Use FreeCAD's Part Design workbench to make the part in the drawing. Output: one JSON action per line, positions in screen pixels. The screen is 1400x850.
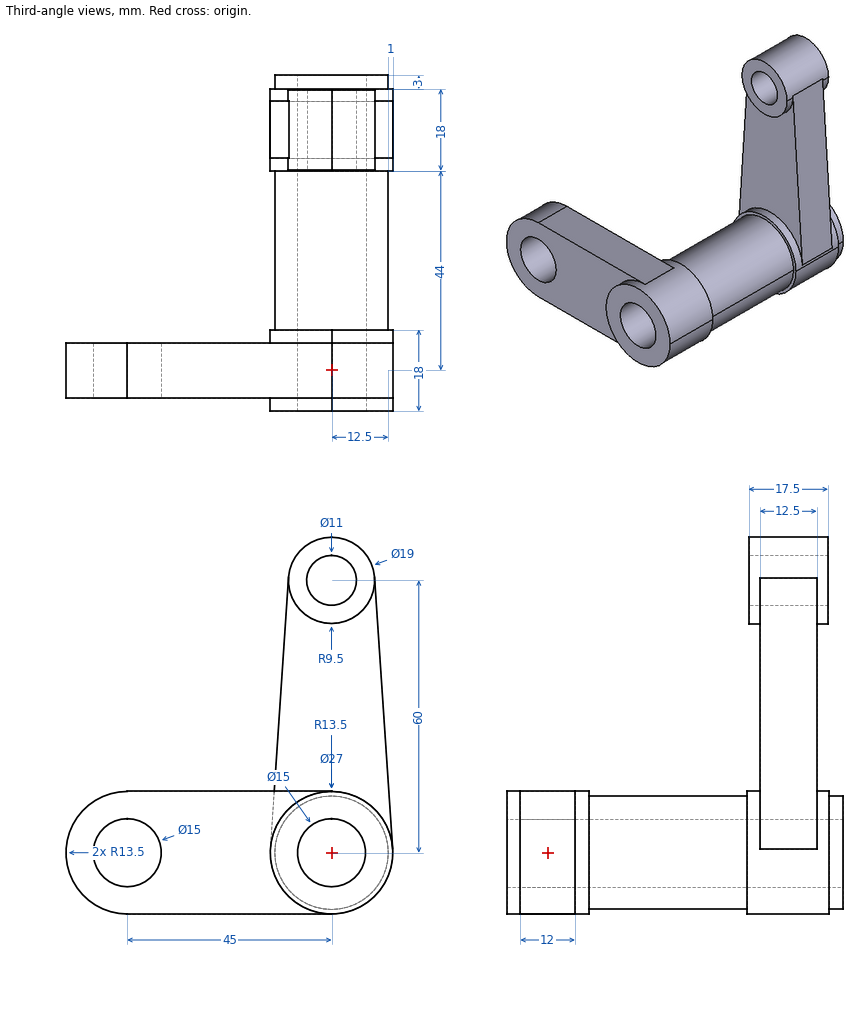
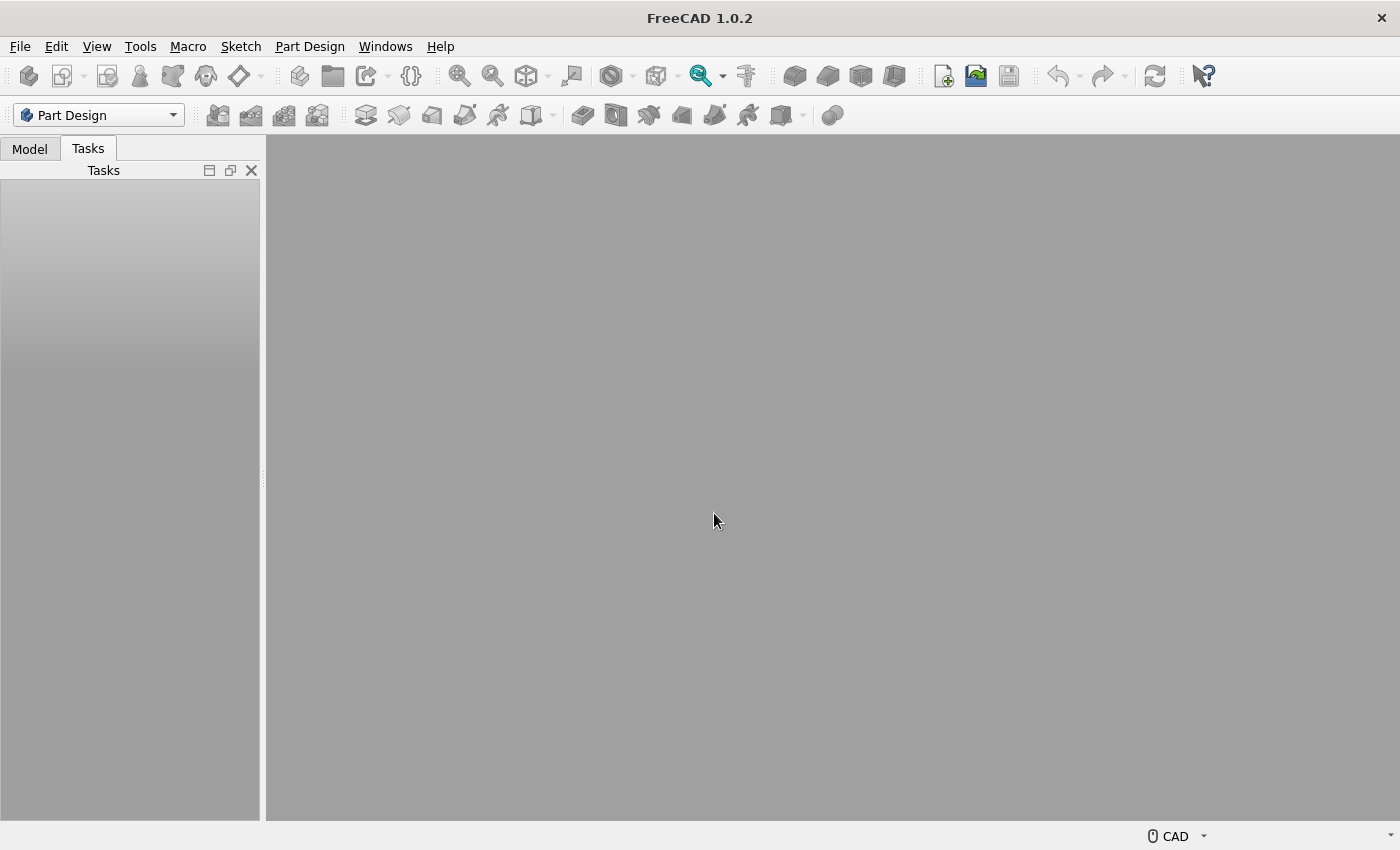
{"action": "left_click", "coordinate": [943, 76]}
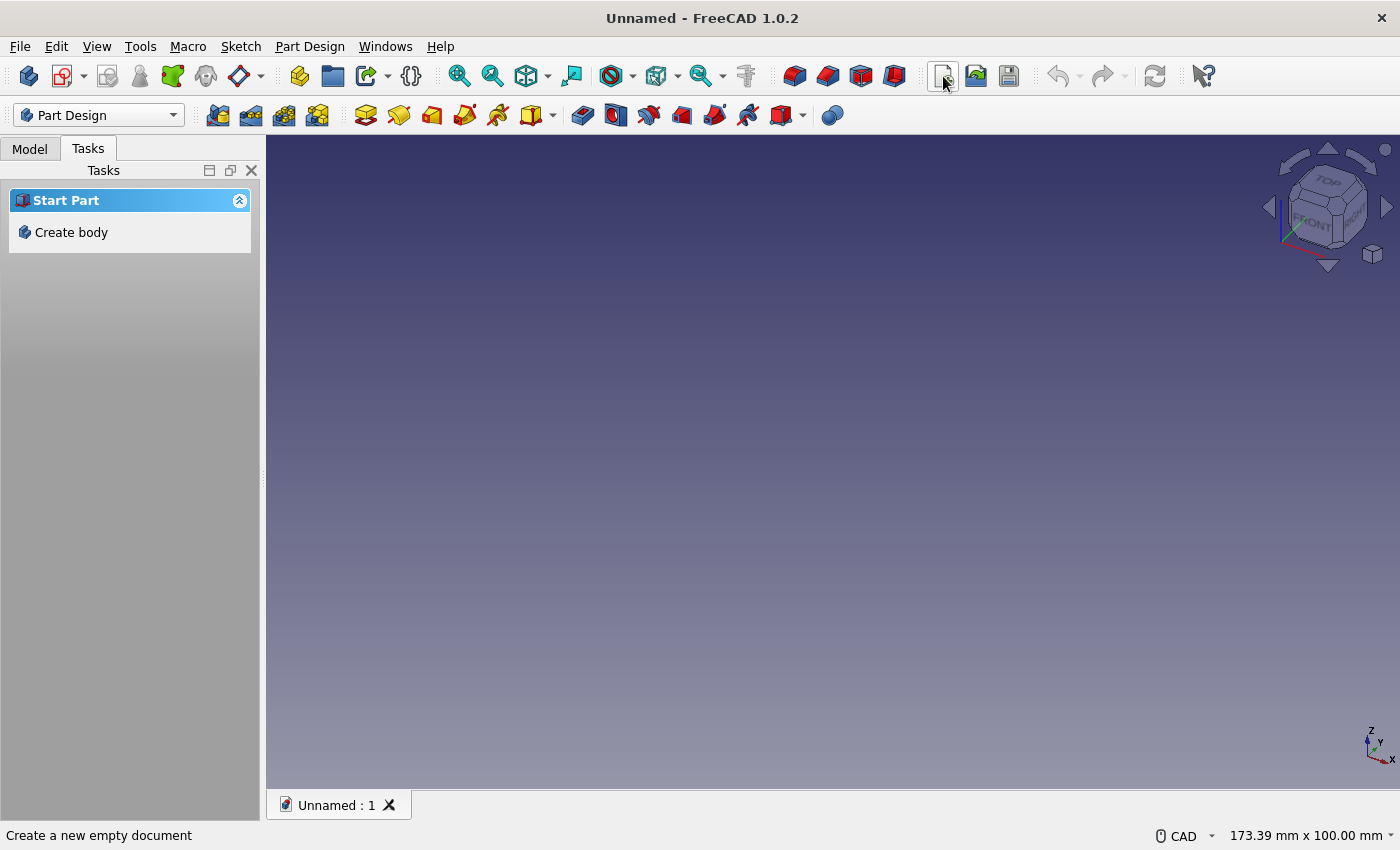
{"action": "left_click", "coordinate": [62, 76]}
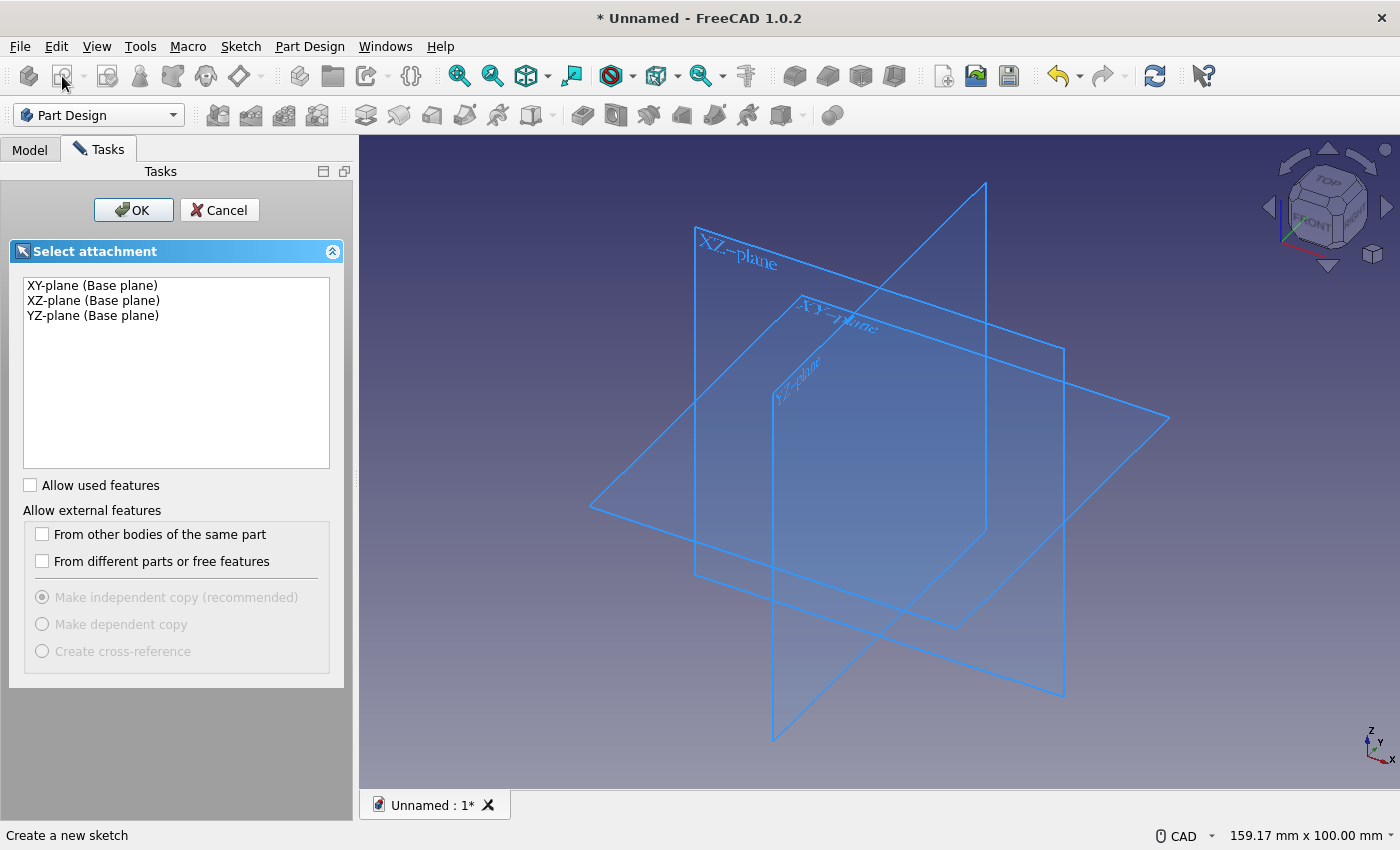
{"action": "left_click", "coordinate": [84, 300]}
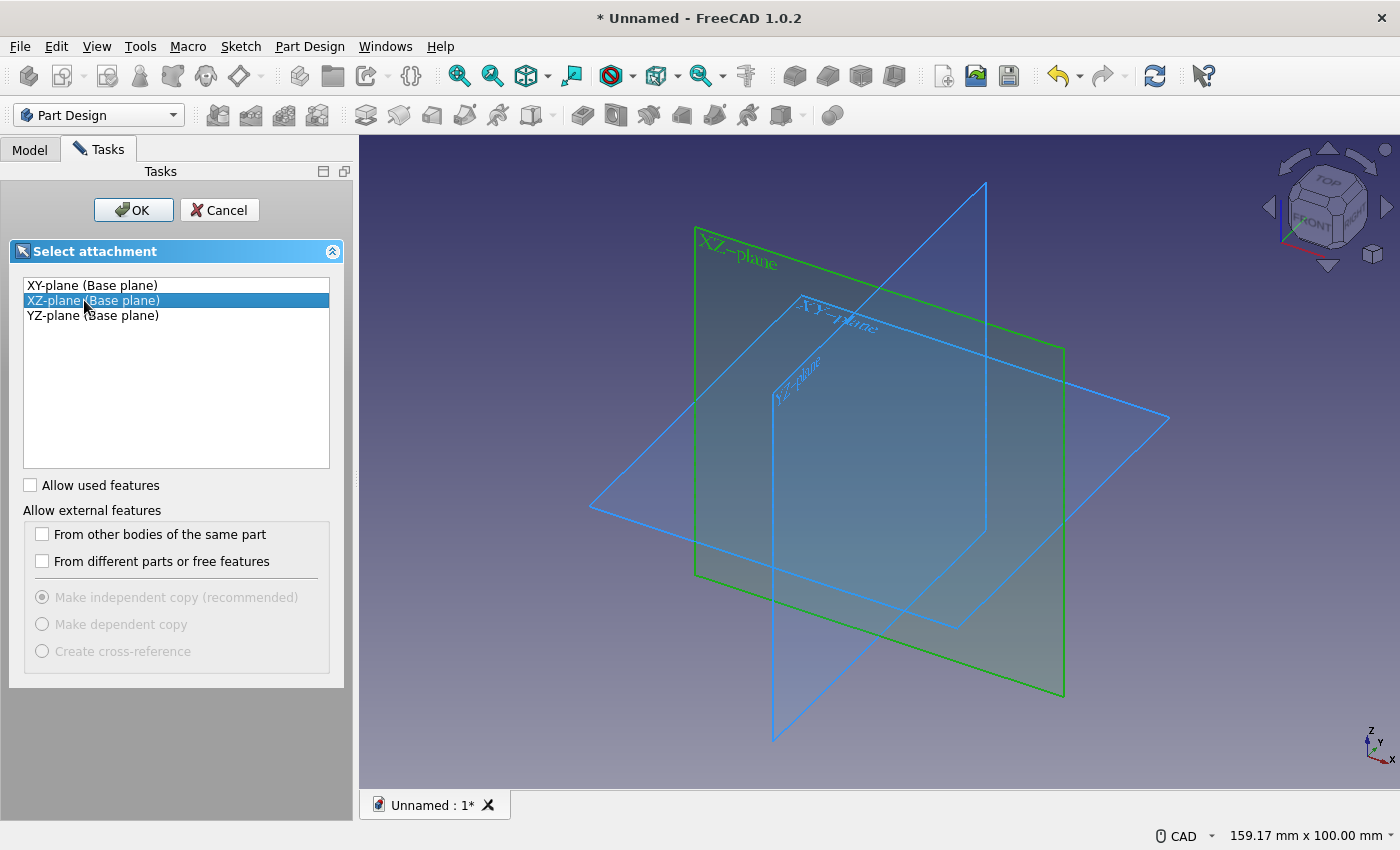
{"action": "left_click", "coordinate": [134, 210]}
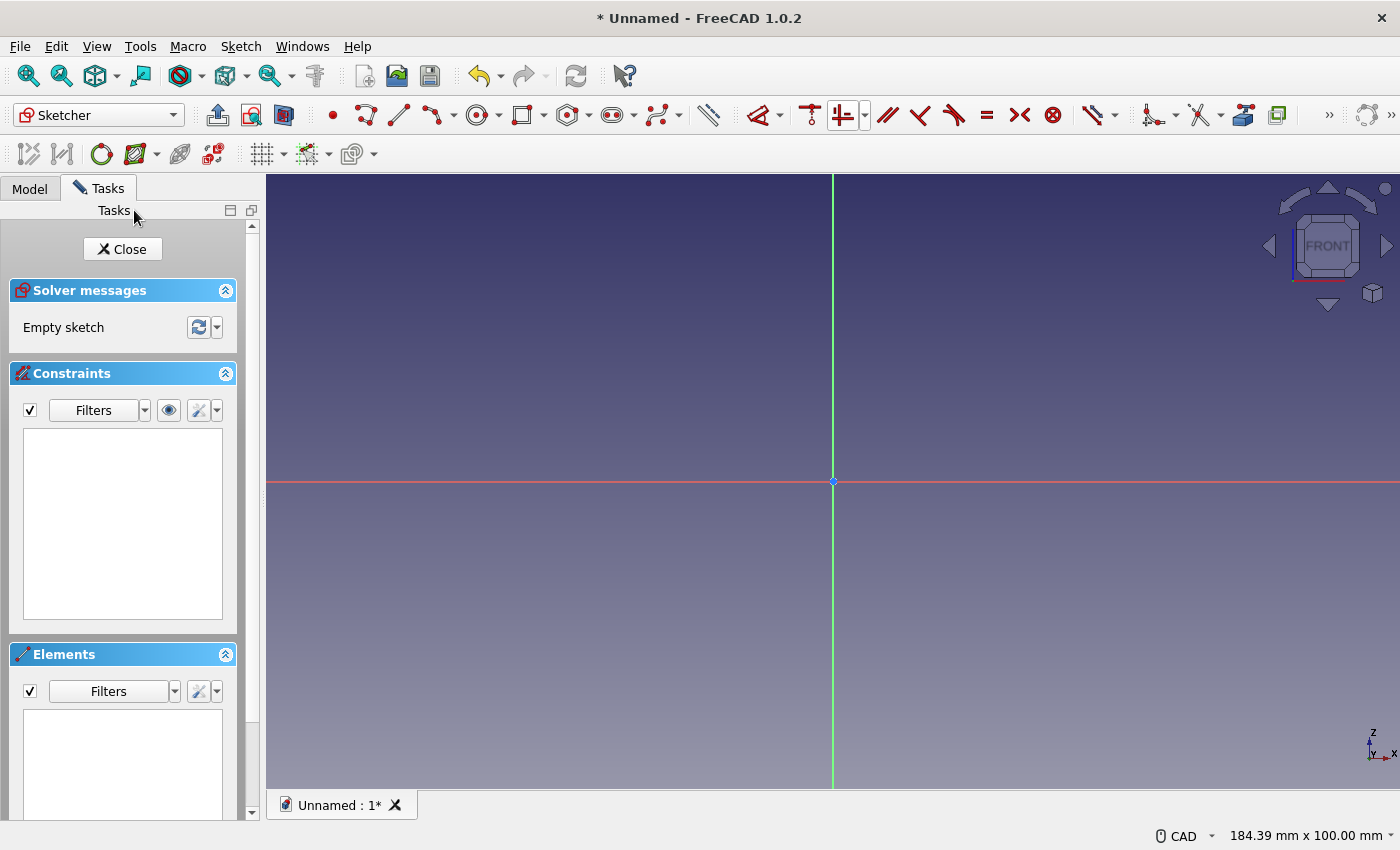
{"action": "scroll", "coordinate": [553, 482], "scroll_direction": "up", "scroll_amount": 2}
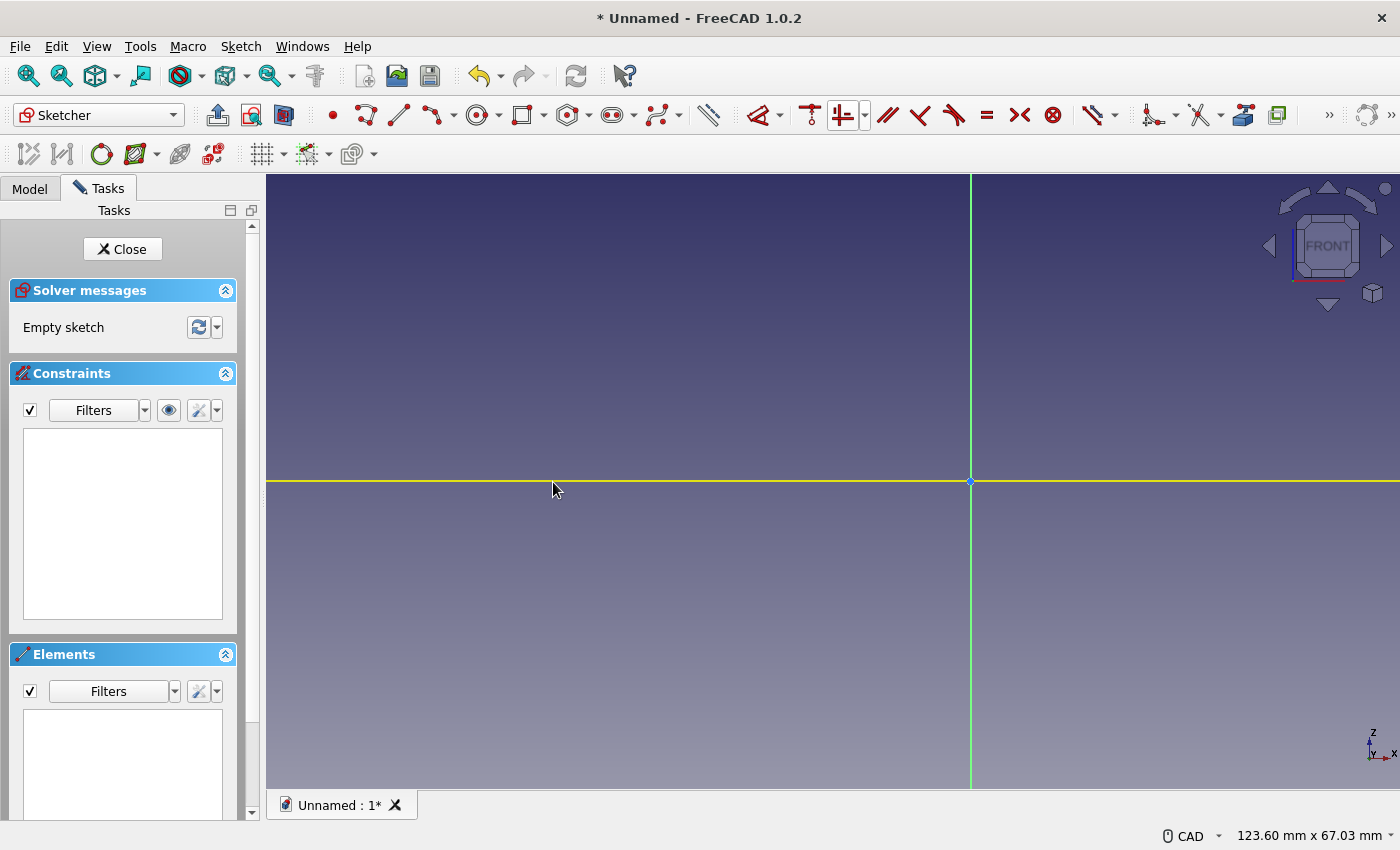
{"action": "key", "text": "g s"}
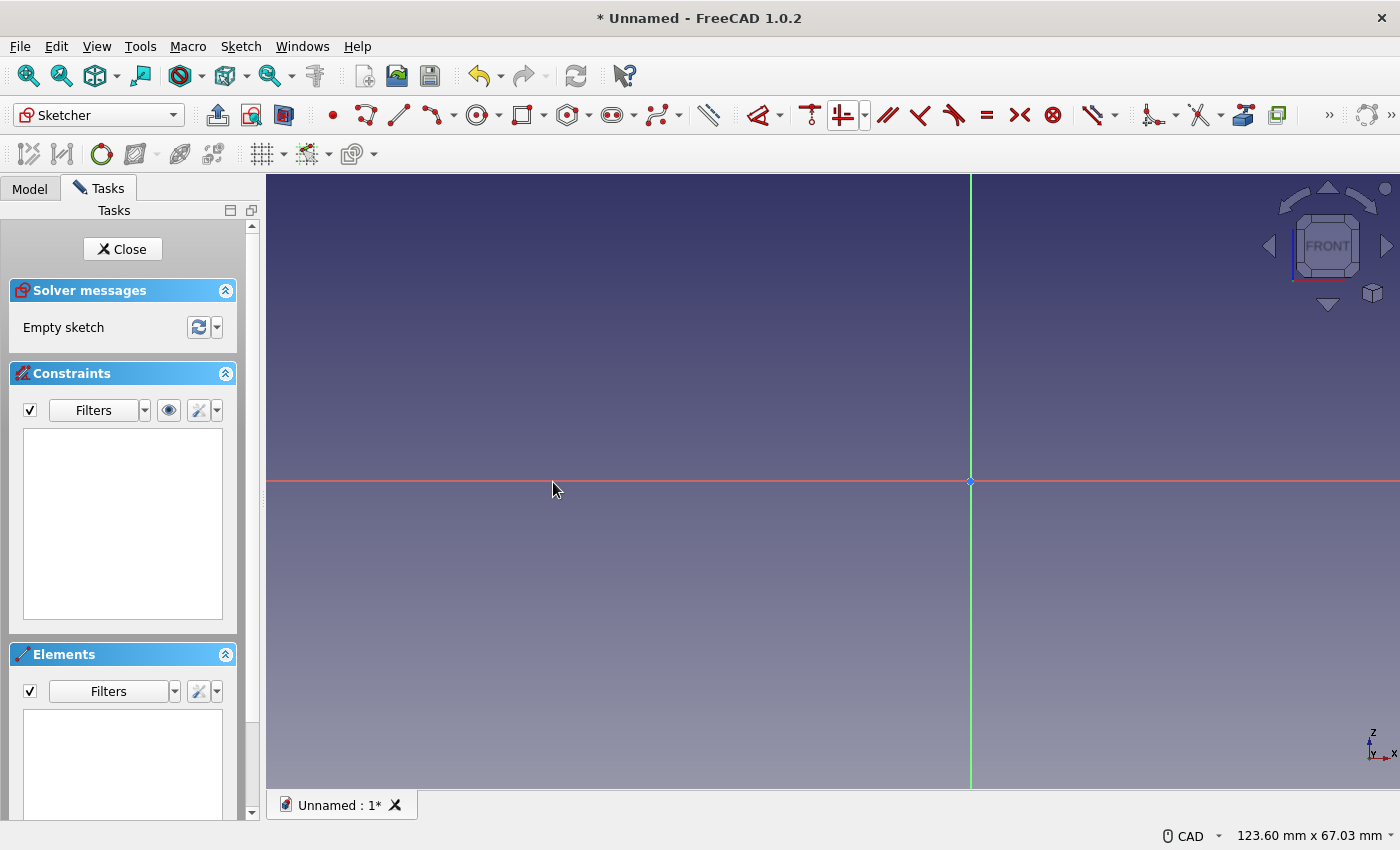
{"action": "left_click", "coordinate": [971, 481]}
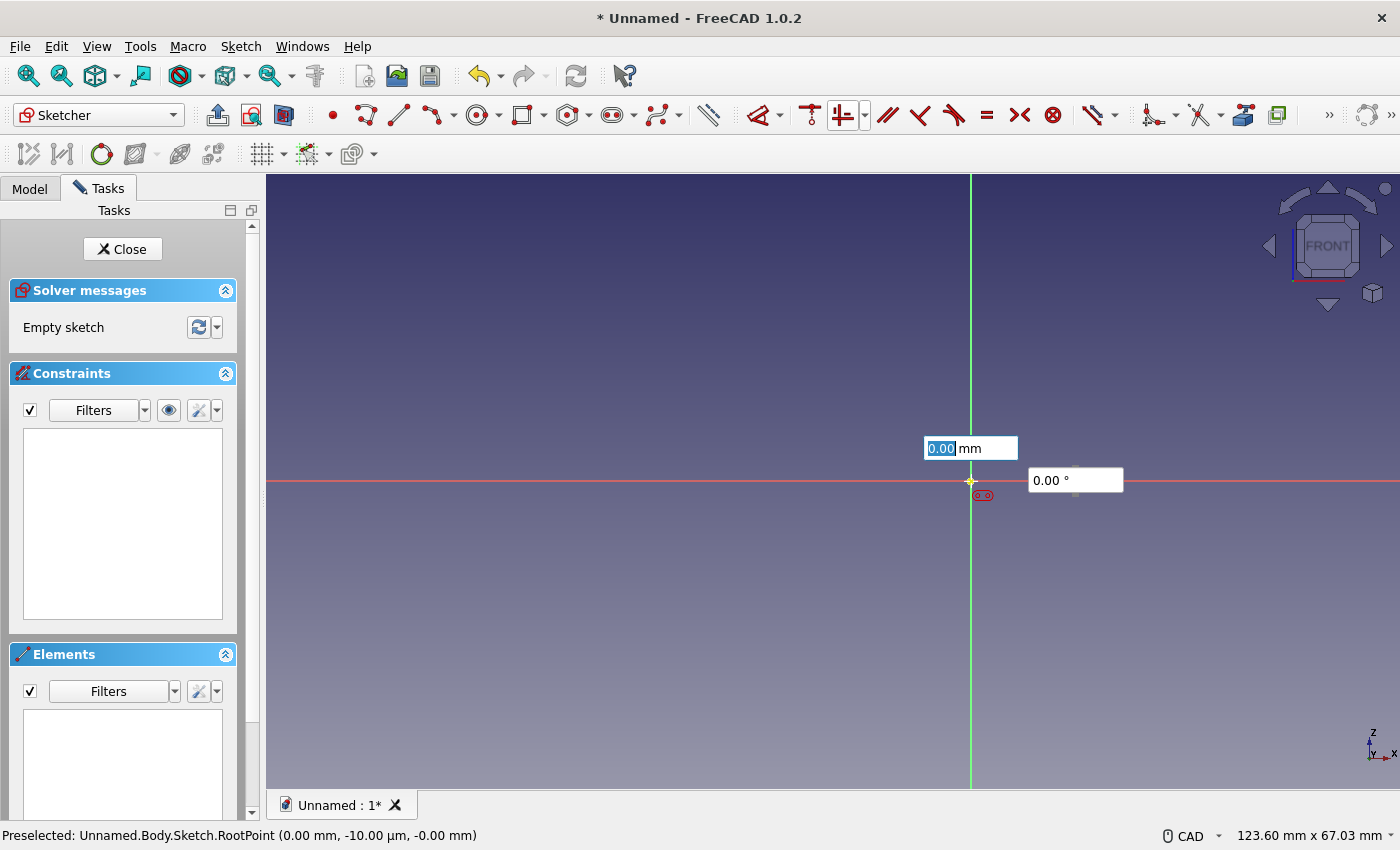
{"action": "left_click", "coordinate": [558, 472]}